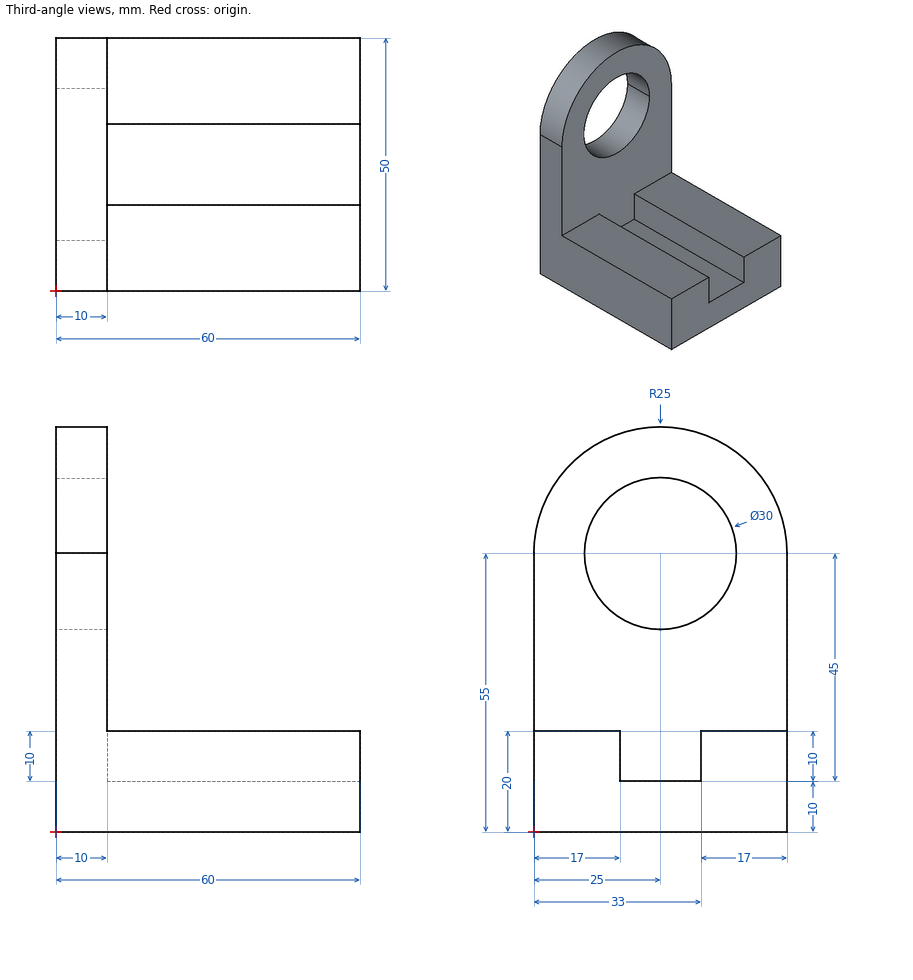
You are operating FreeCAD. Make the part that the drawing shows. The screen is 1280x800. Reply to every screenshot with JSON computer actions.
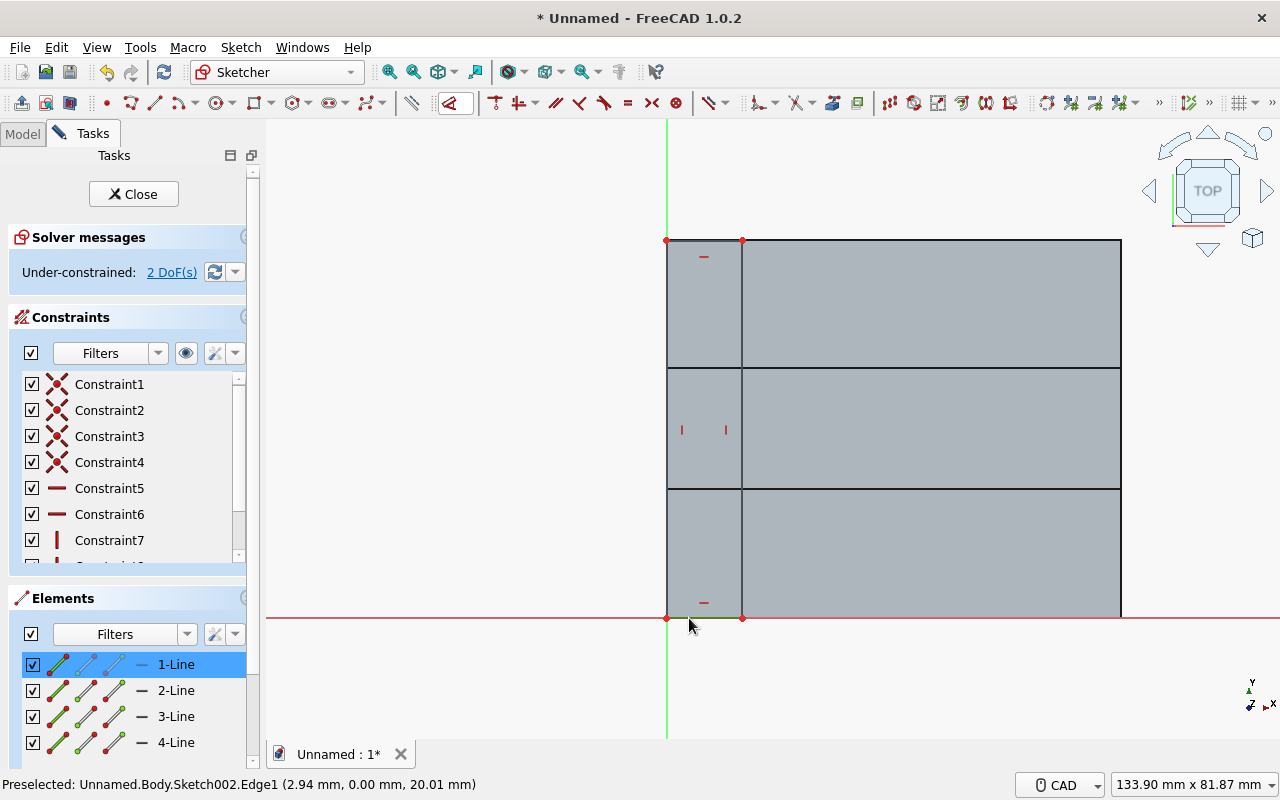
{"action": "key", "text": "l"}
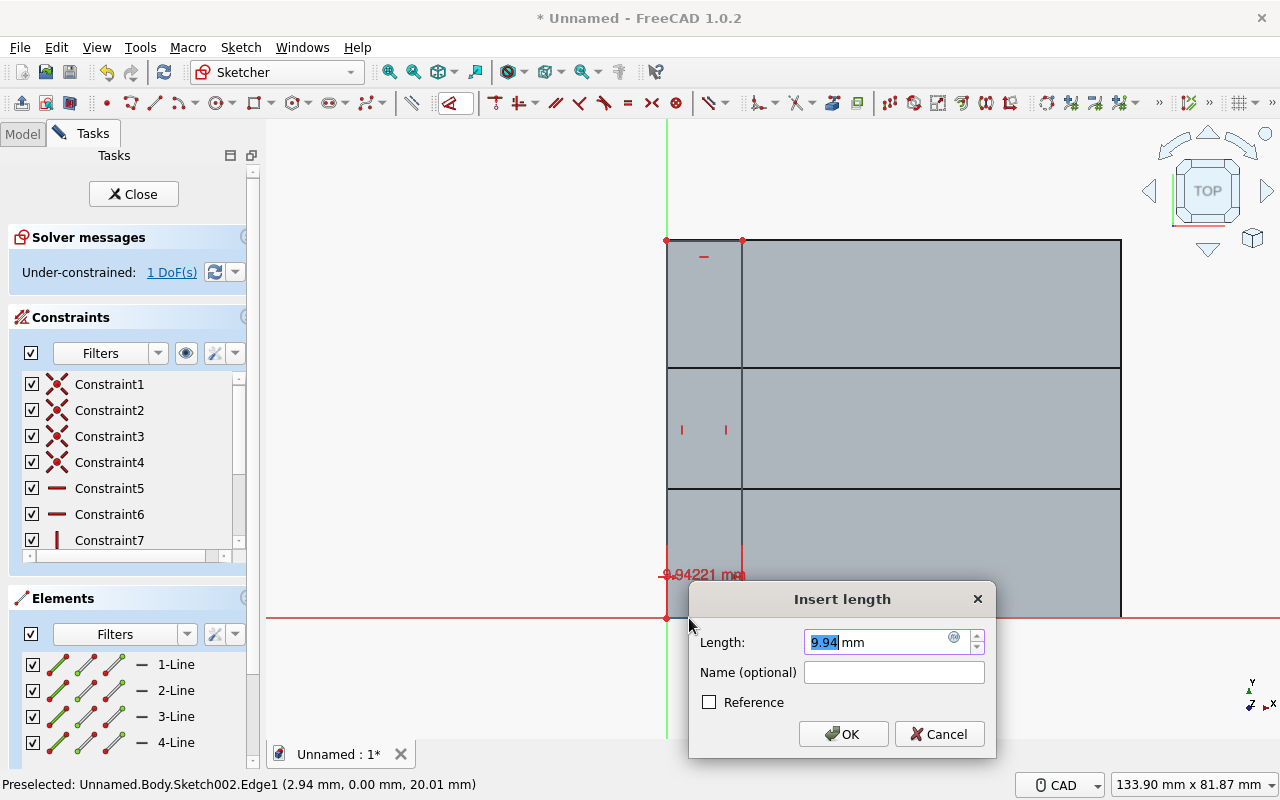
{"action": "type", "text": "10"}
{"action": "key", "text": "Return"}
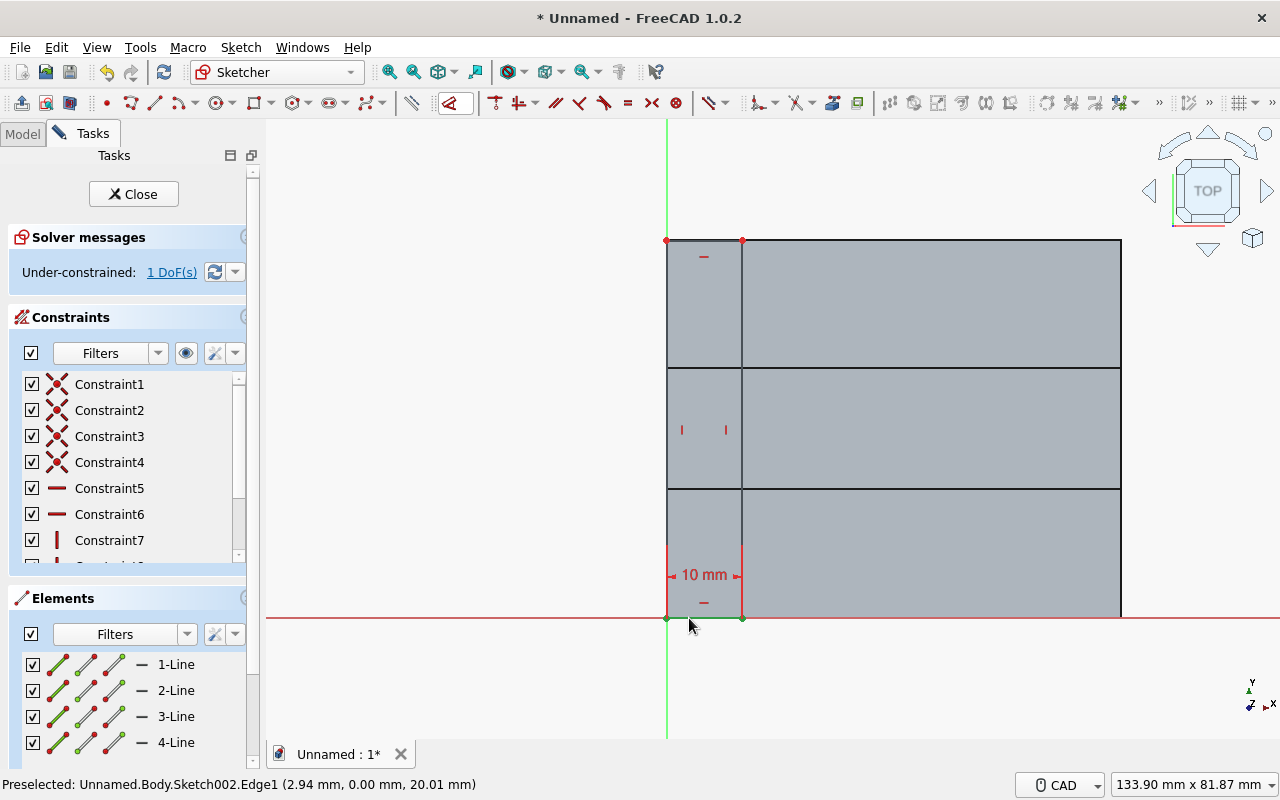
{"action": "left_click", "coordinate": [742, 505]}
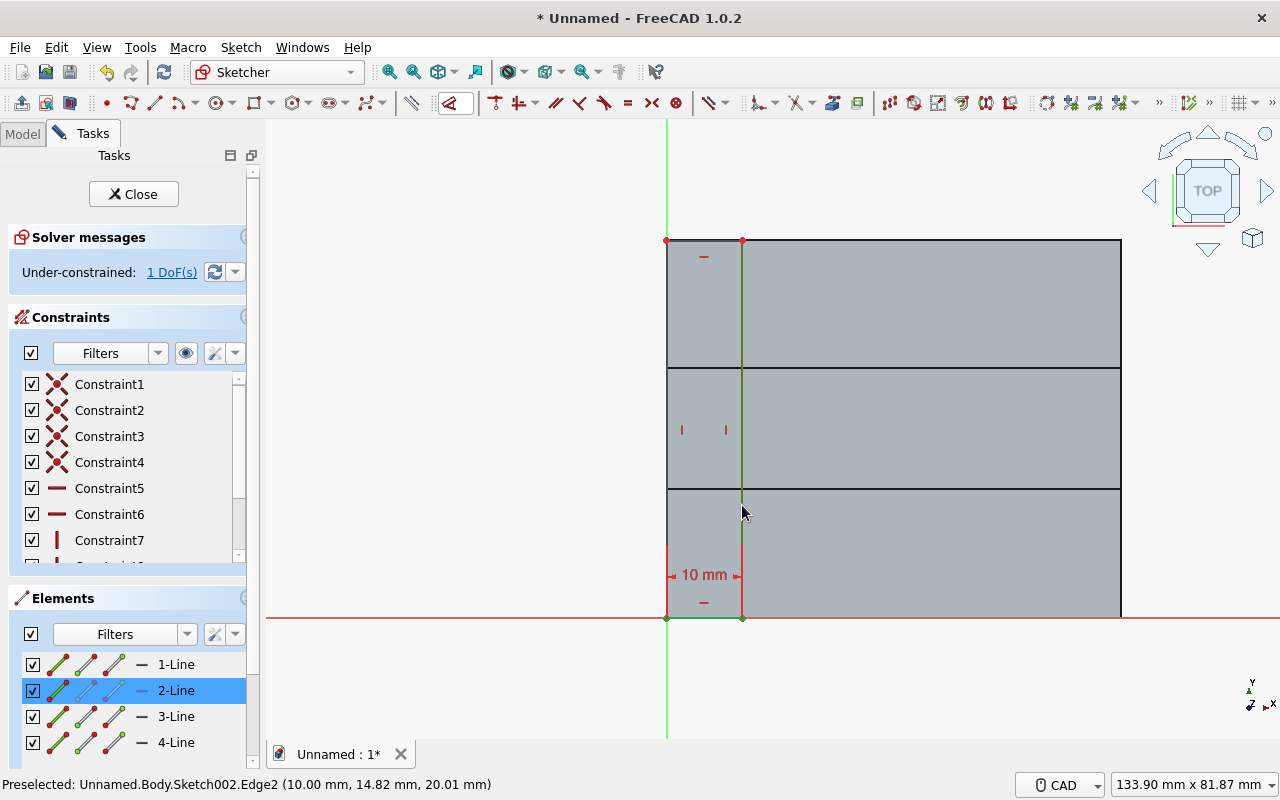
{"action": "left_click", "coordinate": [468, 104]}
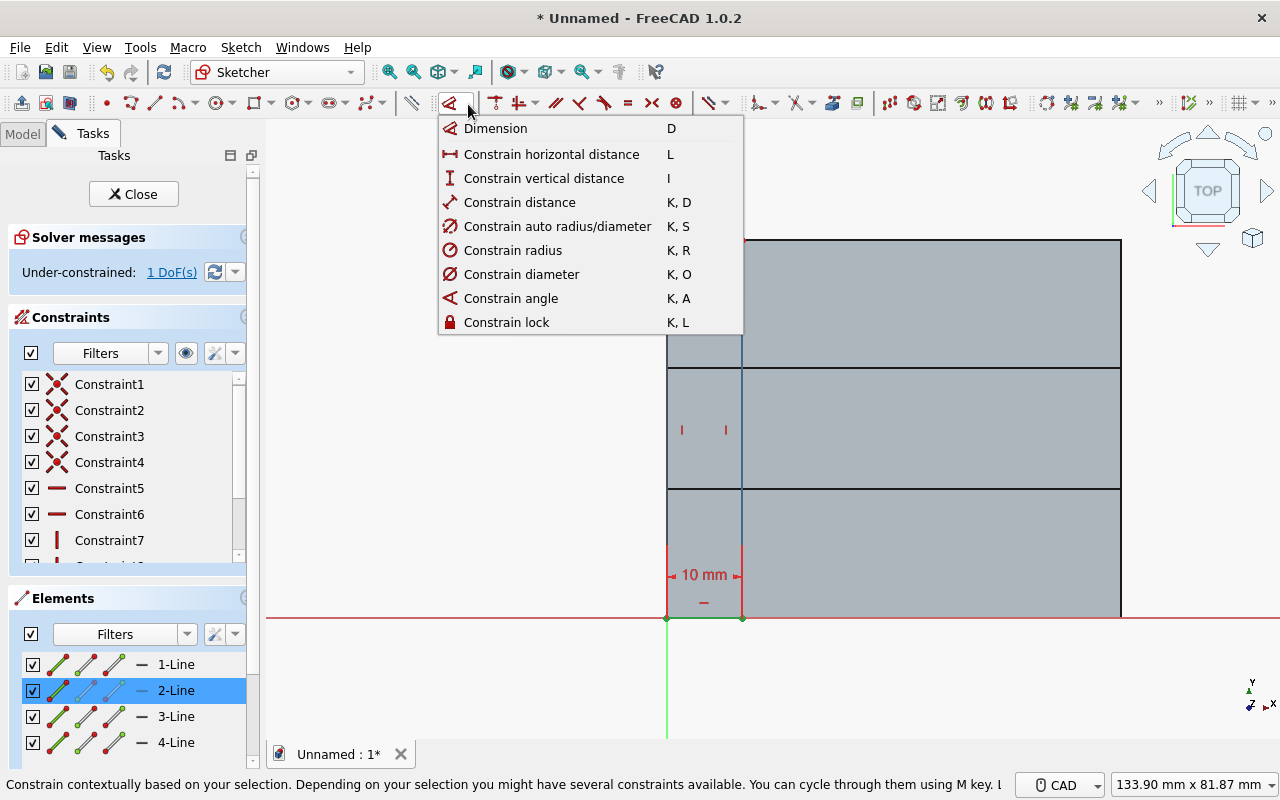
{"action": "left_click", "coordinate": [591, 178]}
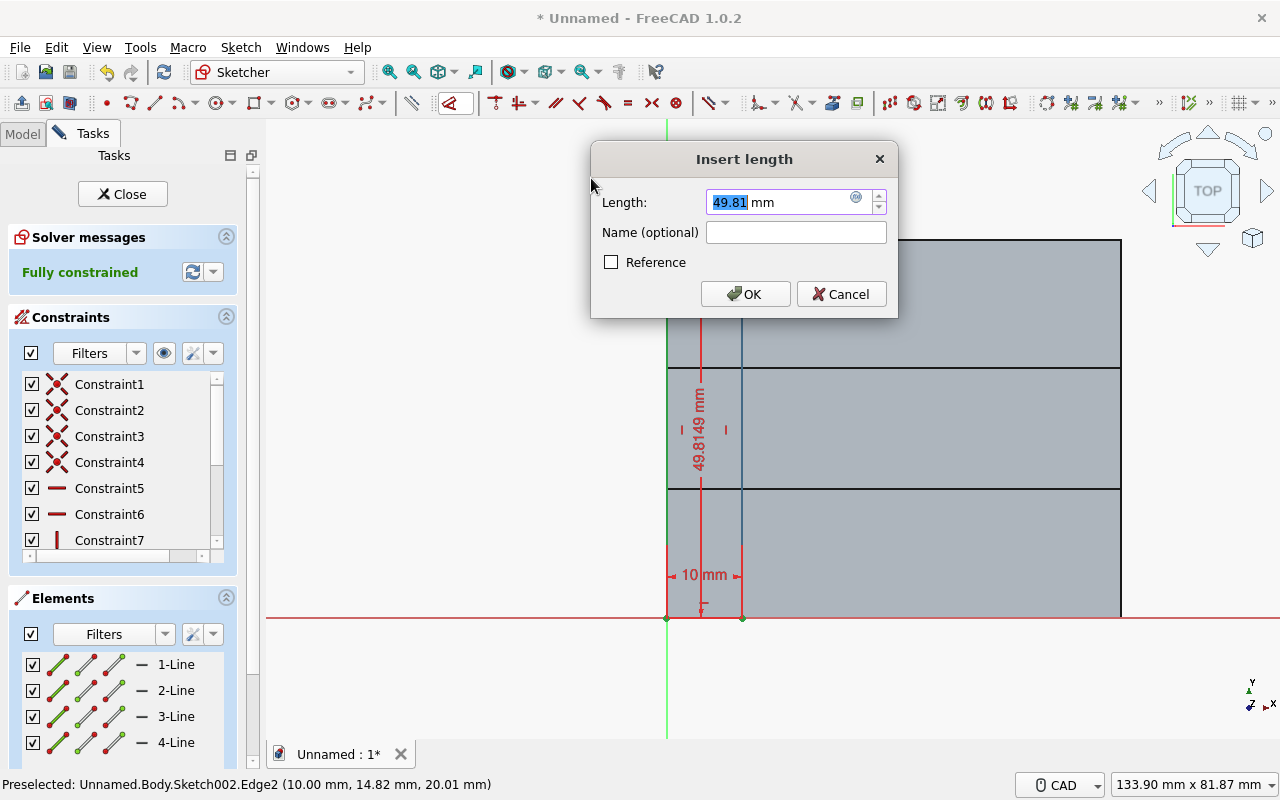
{"action": "type", "text": "50"}
{"action": "key", "text": "Return"}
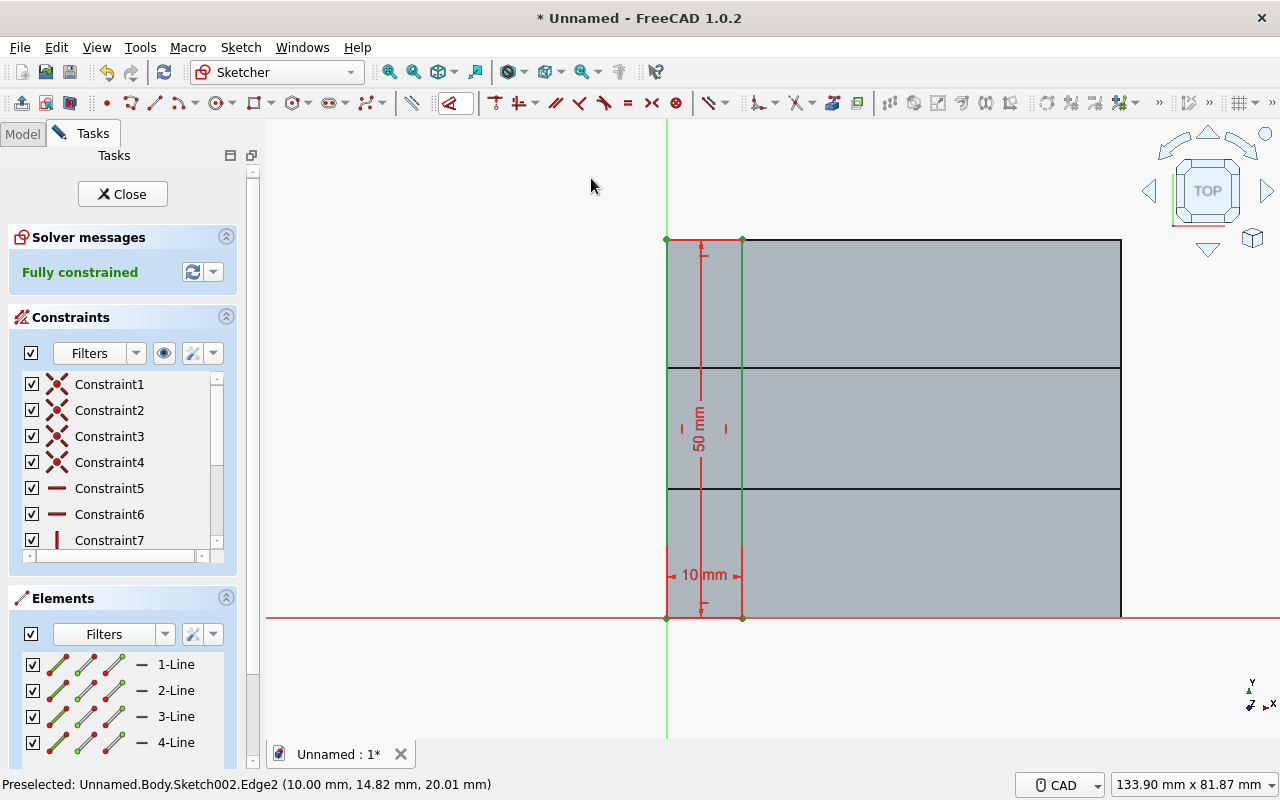
{"action": "left_click", "coordinate": [123, 194]}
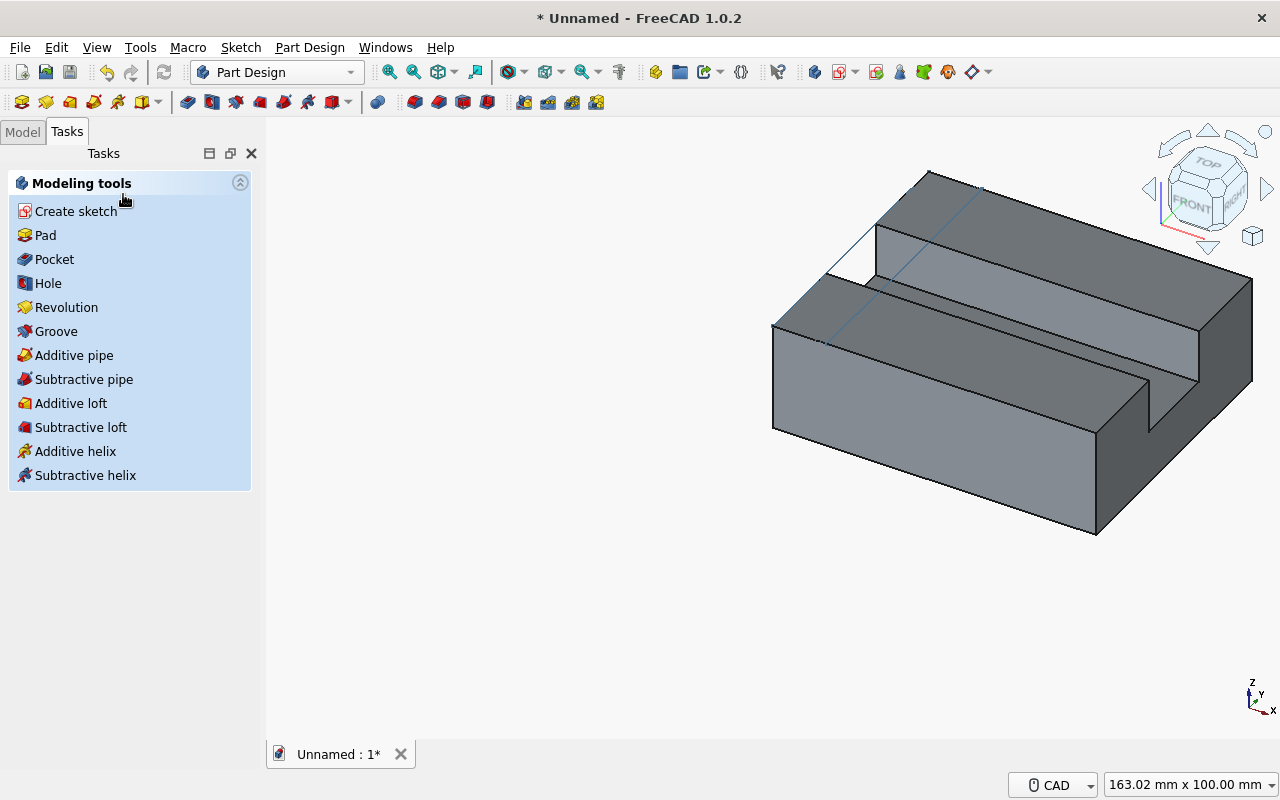
{"action": "left_click", "coordinate": [188, 102]}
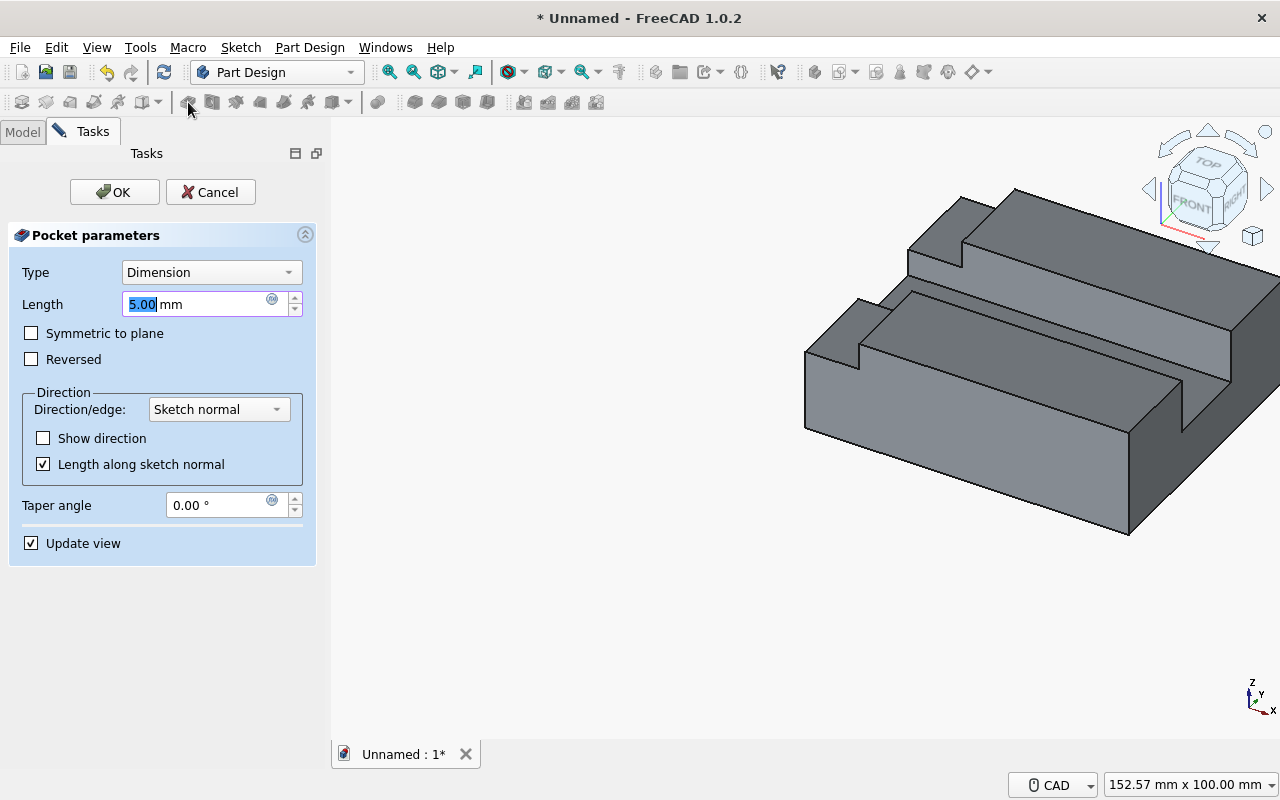
{"action": "type", "text": "10"}
{"action": "key", "text": "Tab"}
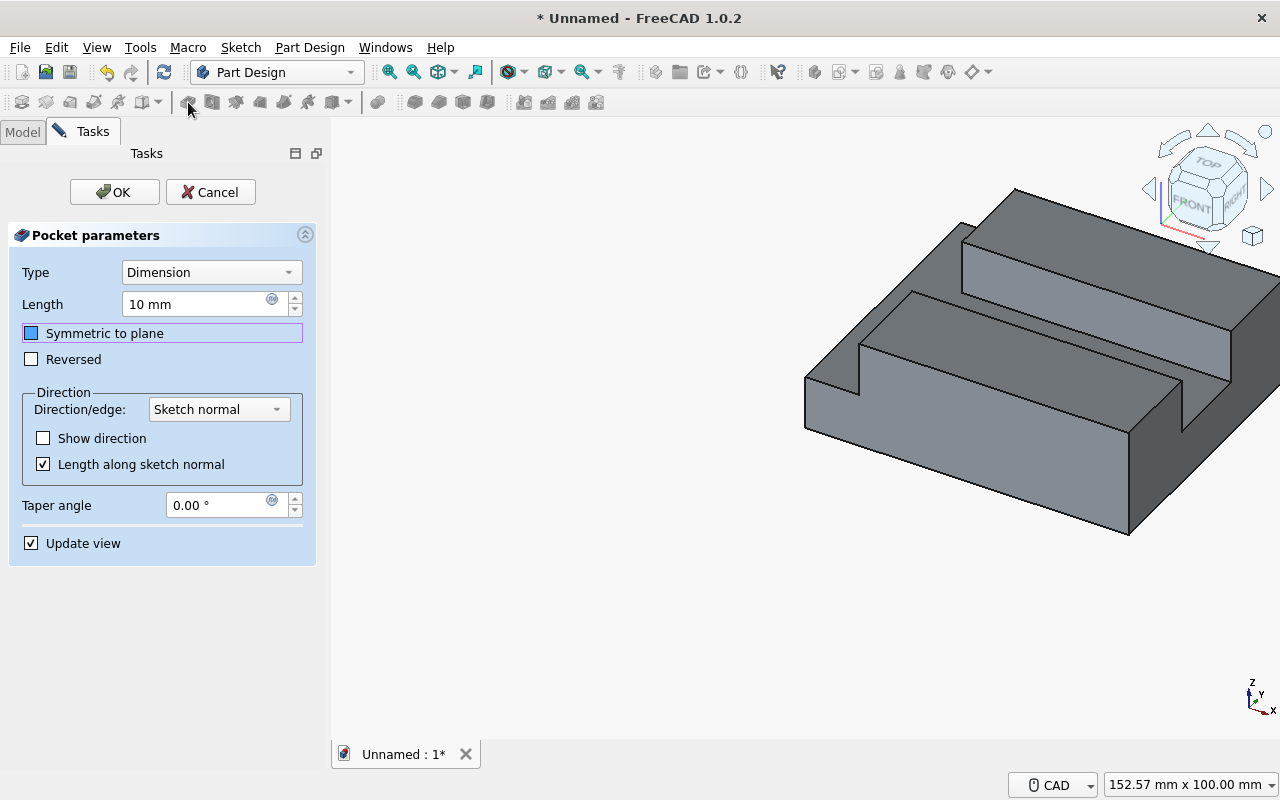
{"action": "left_click", "coordinate": [115, 192]}